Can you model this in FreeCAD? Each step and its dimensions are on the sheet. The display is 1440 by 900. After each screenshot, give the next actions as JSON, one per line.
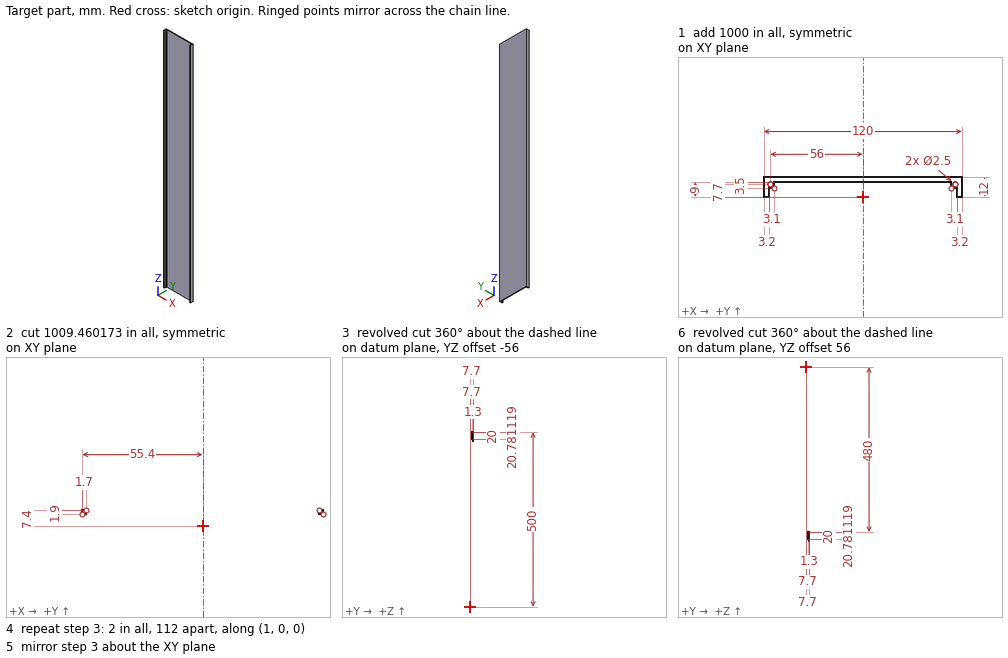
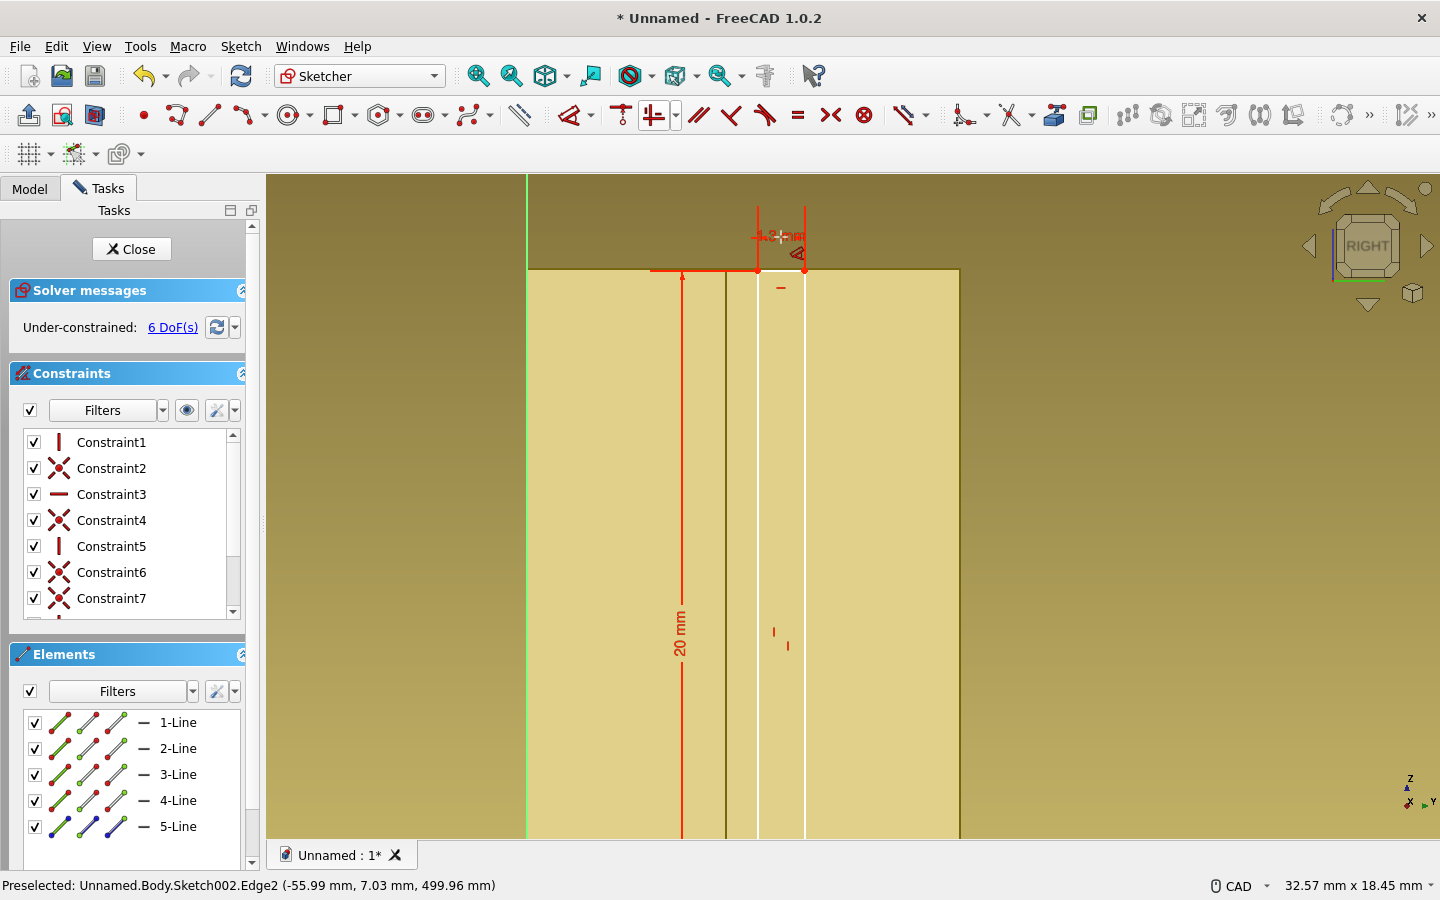
{"action": "scroll", "coordinate": [787, 272], "scroll_direction": "down", "scroll_amount": 4}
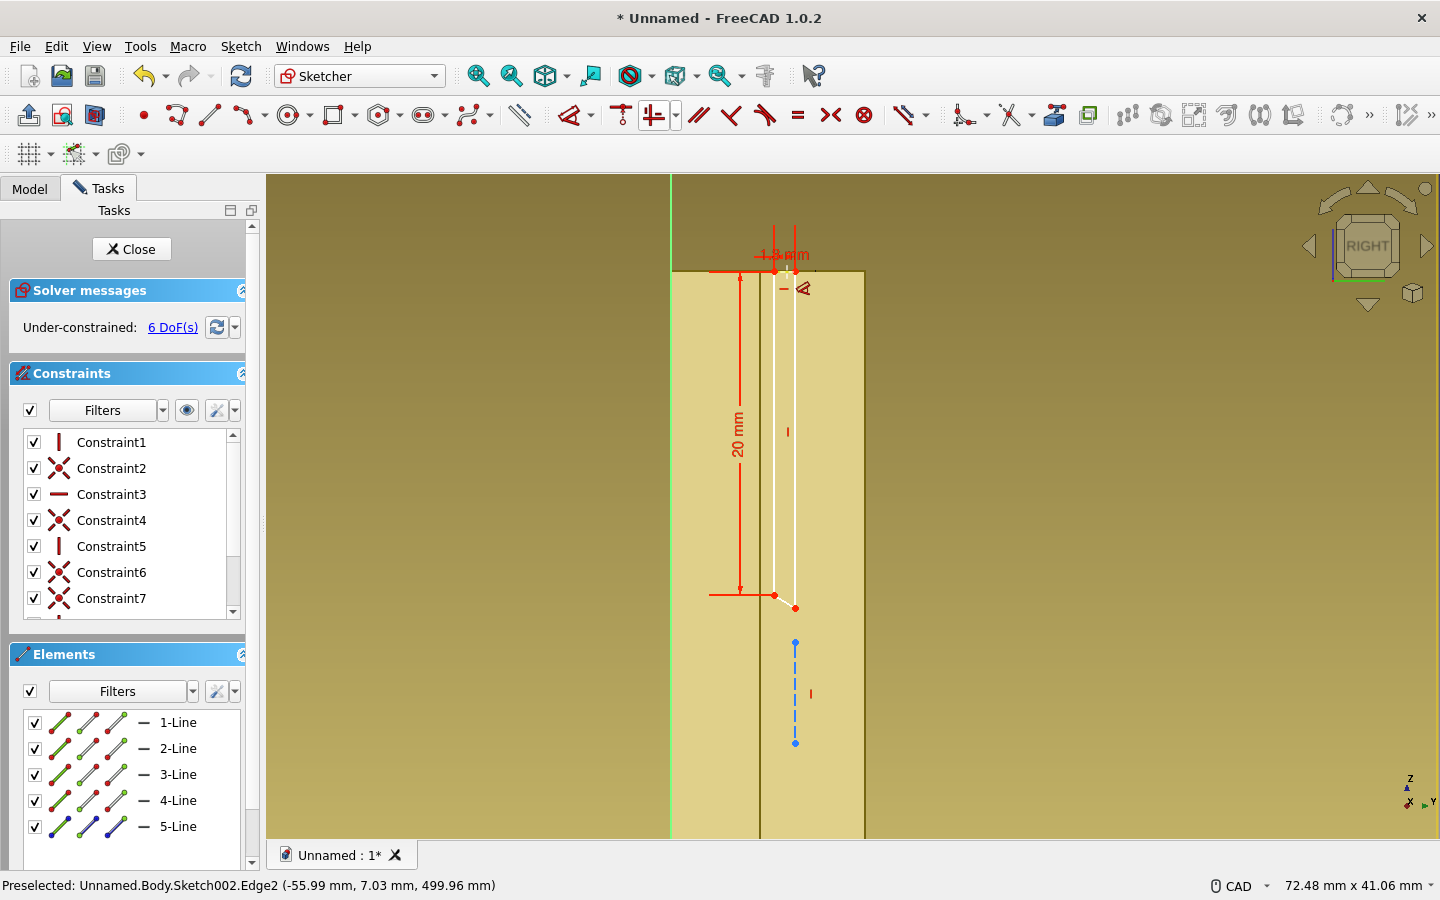
{"action": "left_click", "coordinate": [795, 609]}
{"action": "left_click", "coordinate": [733, 575]}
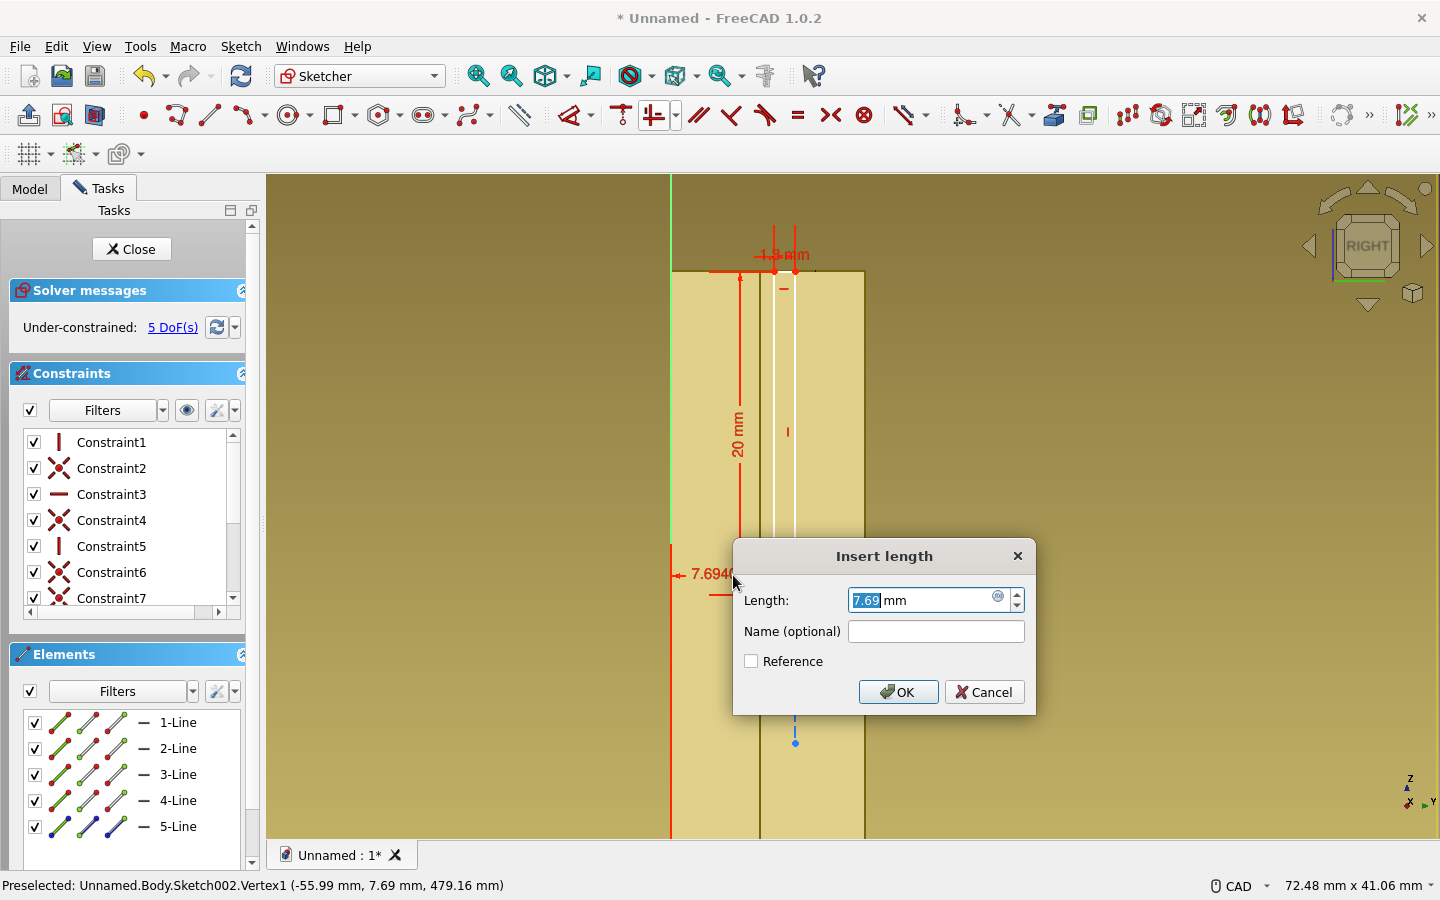
{"action": "type", "text": "7.7"}
{"action": "key", "text": "Return"}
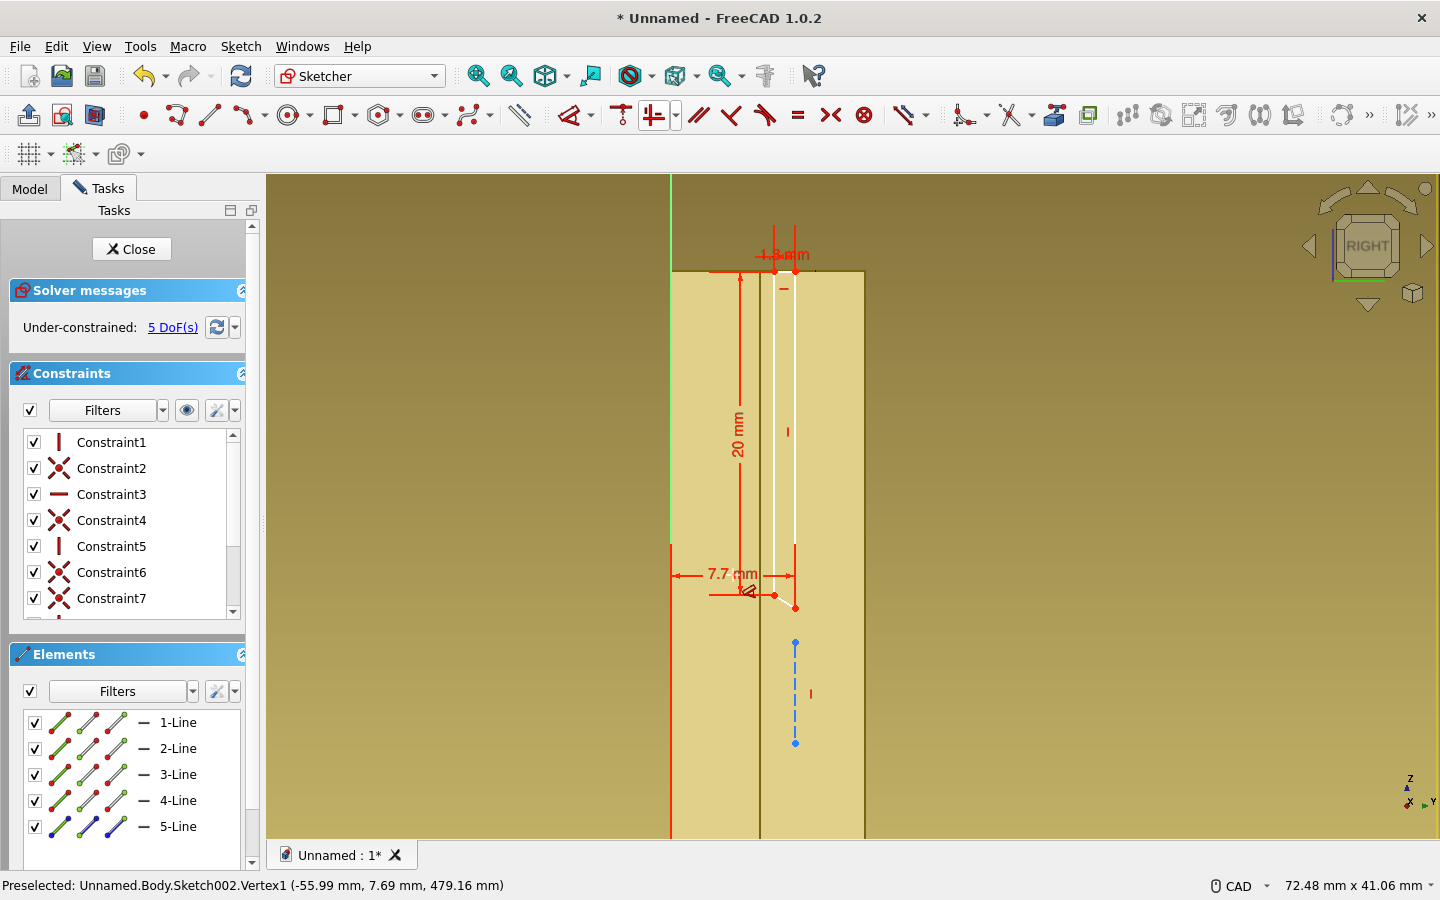
{"action": "left_click", "coordinate": [795, 272]}
{"action": "left_click", "coordinate": [637, 541]}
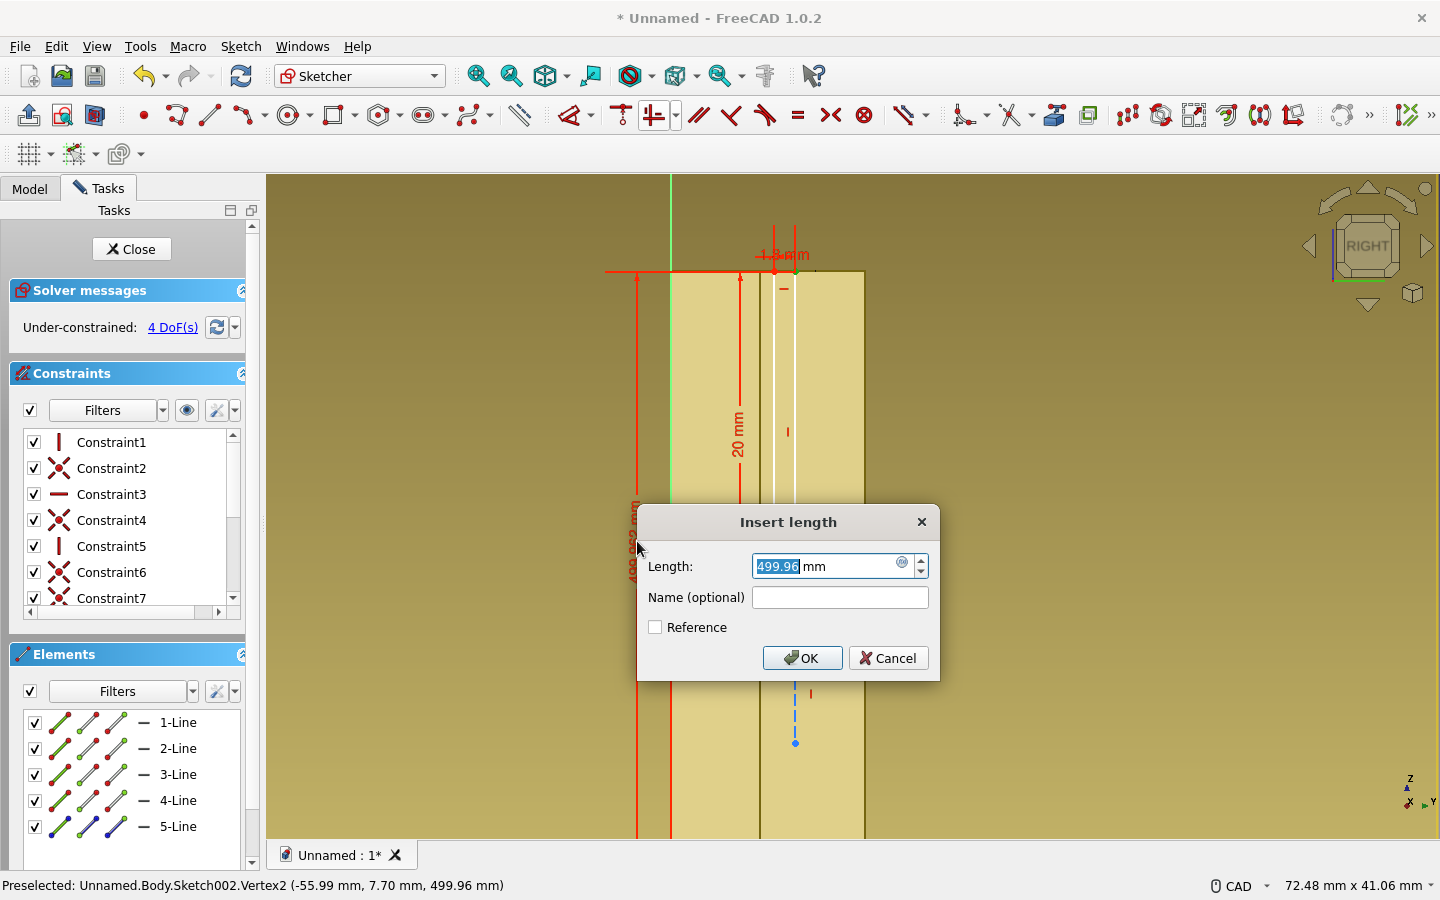
{"action": "type", "text": "500"}
{"action": "key", "text": "Return"}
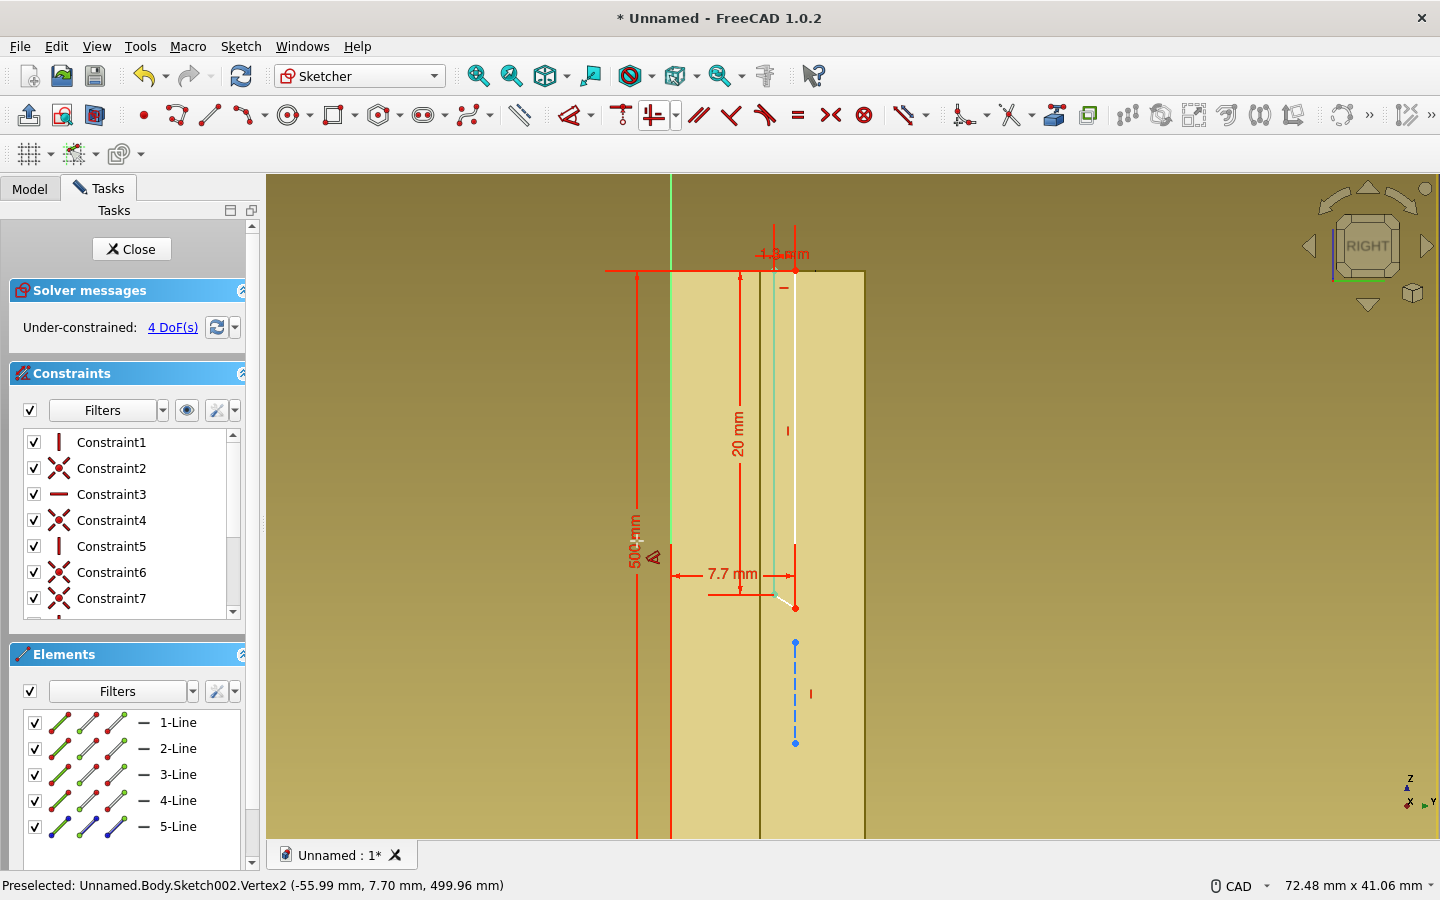
{"action": "left_click", "coordinate": [795, 643]}
{"action": "left_click", "coordinate": [733, 609]}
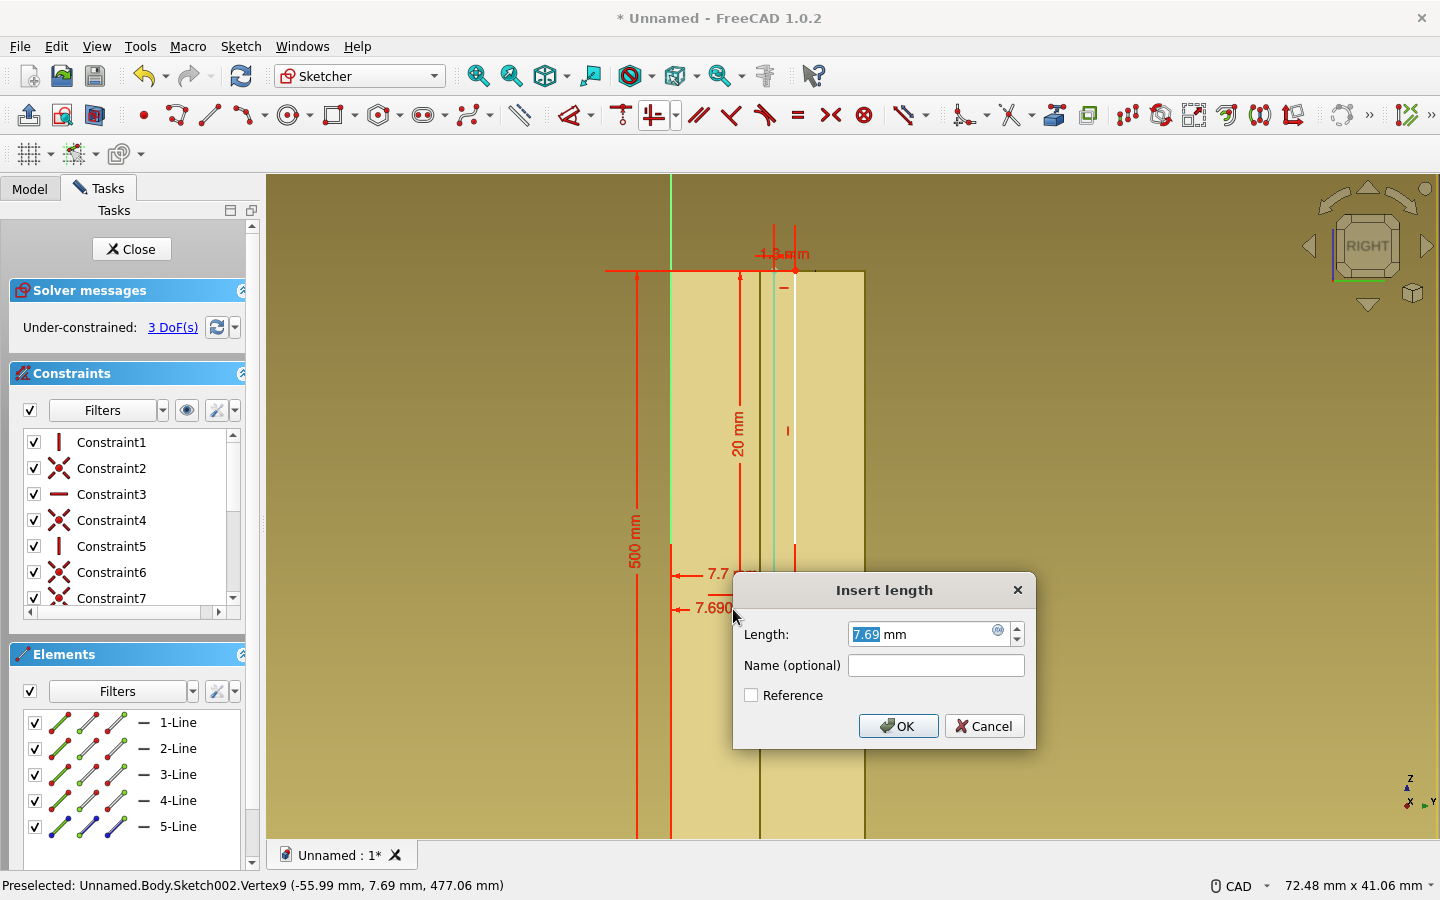
{"action": "type", "text": "7.7"}
{"action": "key", "text": "Return"}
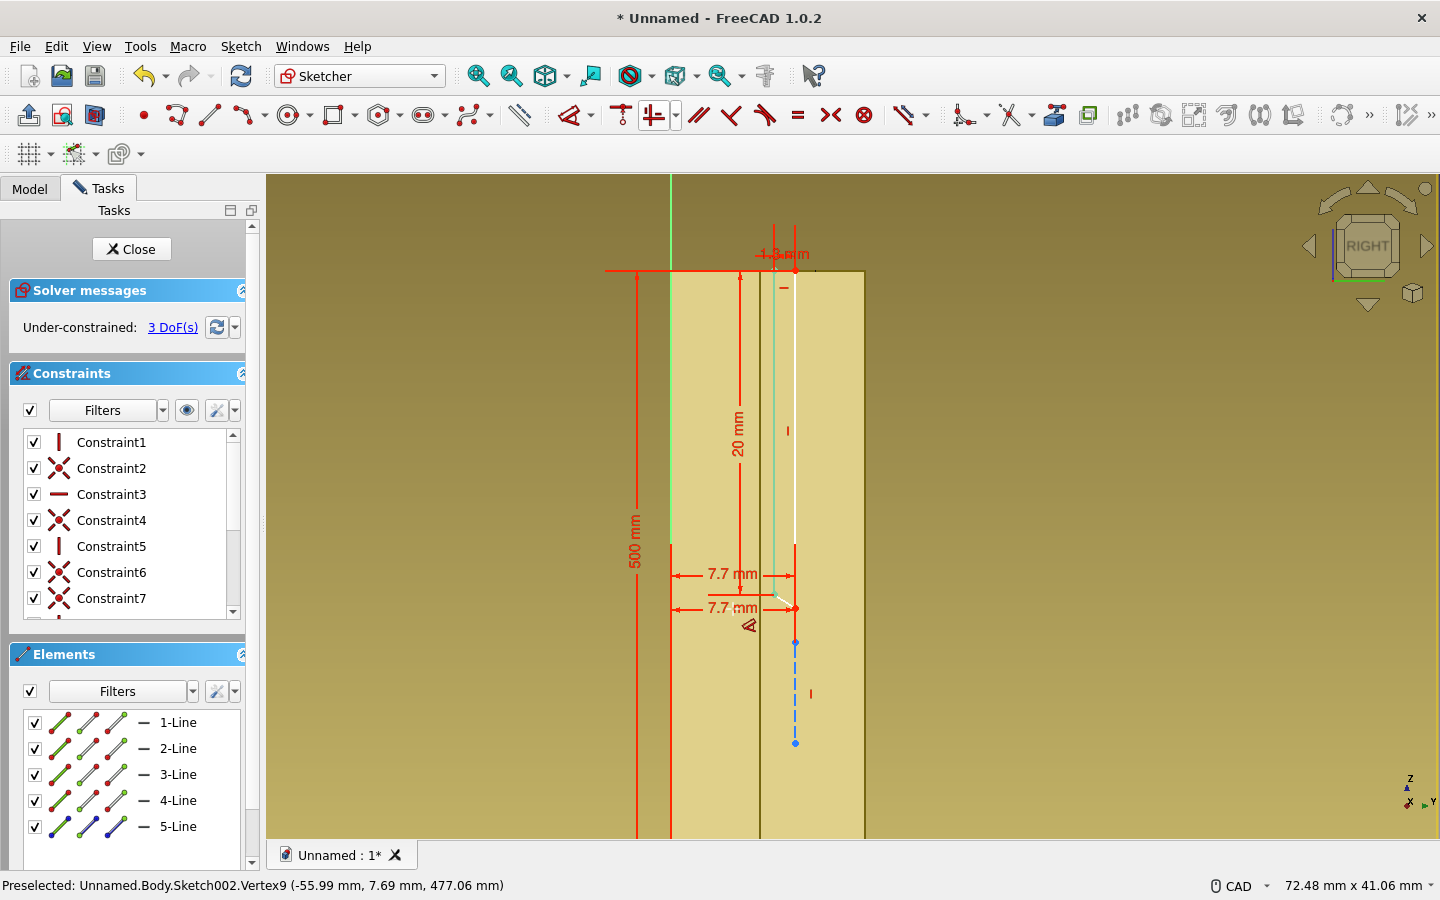
{"action": "left_click", "coordinate": [795, 507]}
{"action": "left_click", "coordinate": [829, 440]}